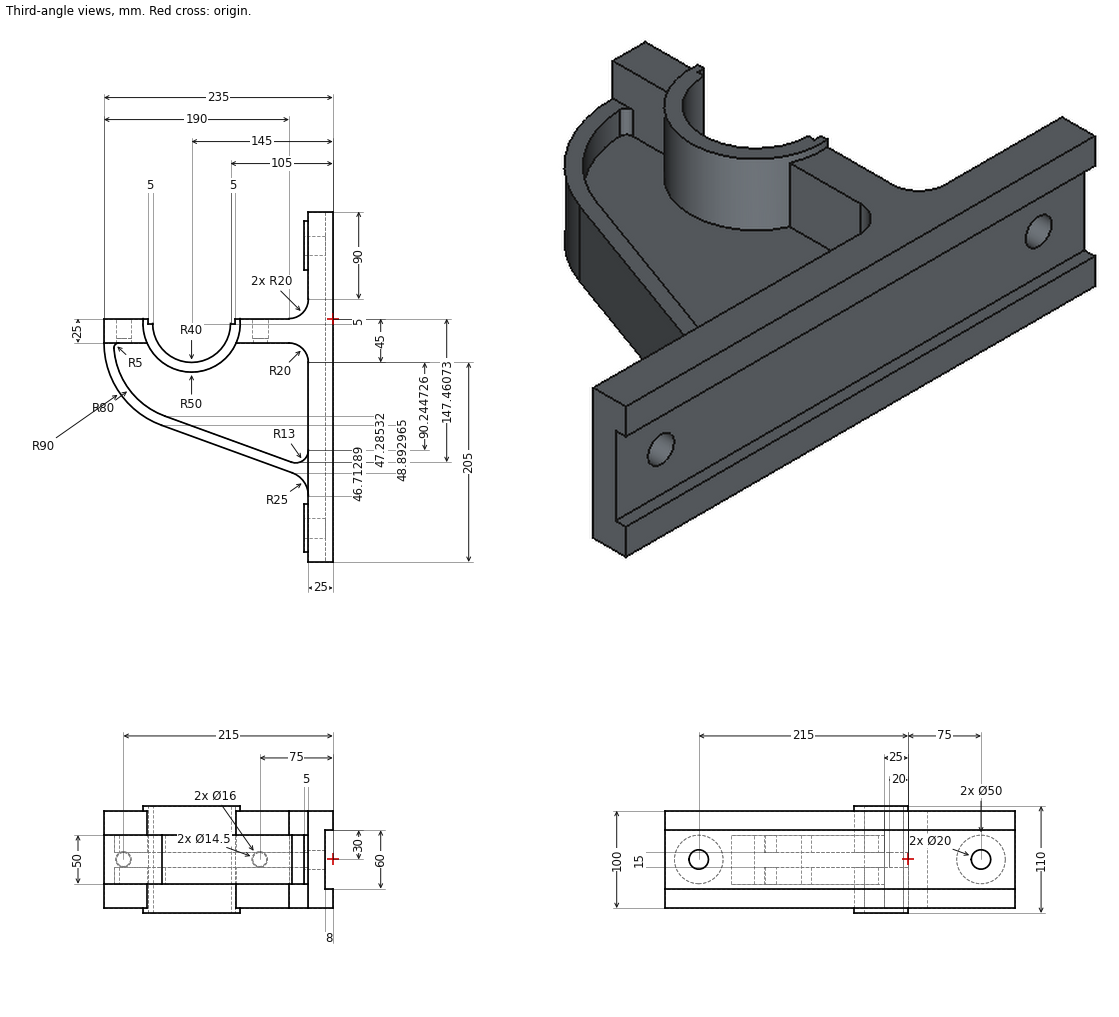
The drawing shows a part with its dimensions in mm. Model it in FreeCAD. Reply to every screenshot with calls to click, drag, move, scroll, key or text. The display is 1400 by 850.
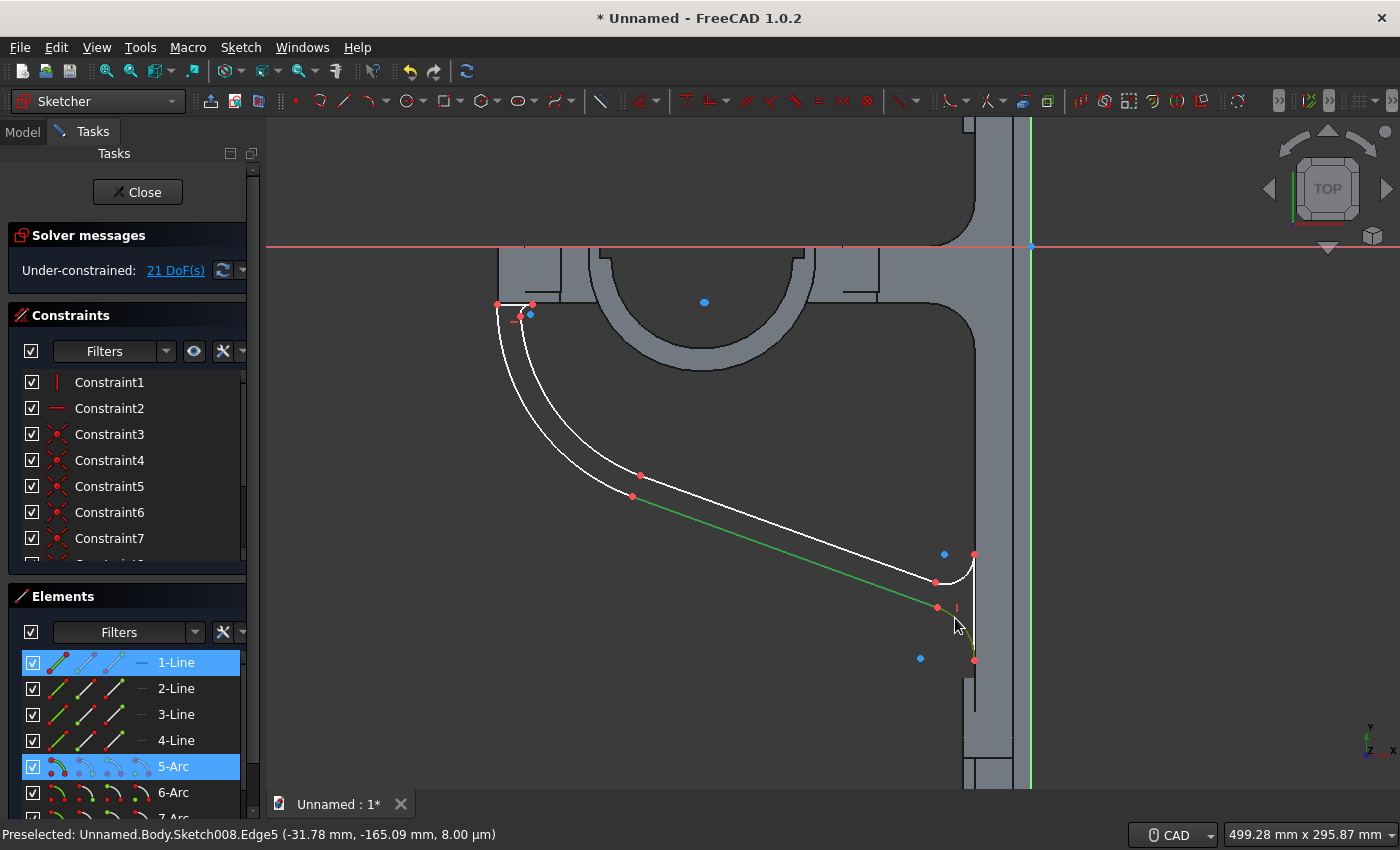
click(796, 102)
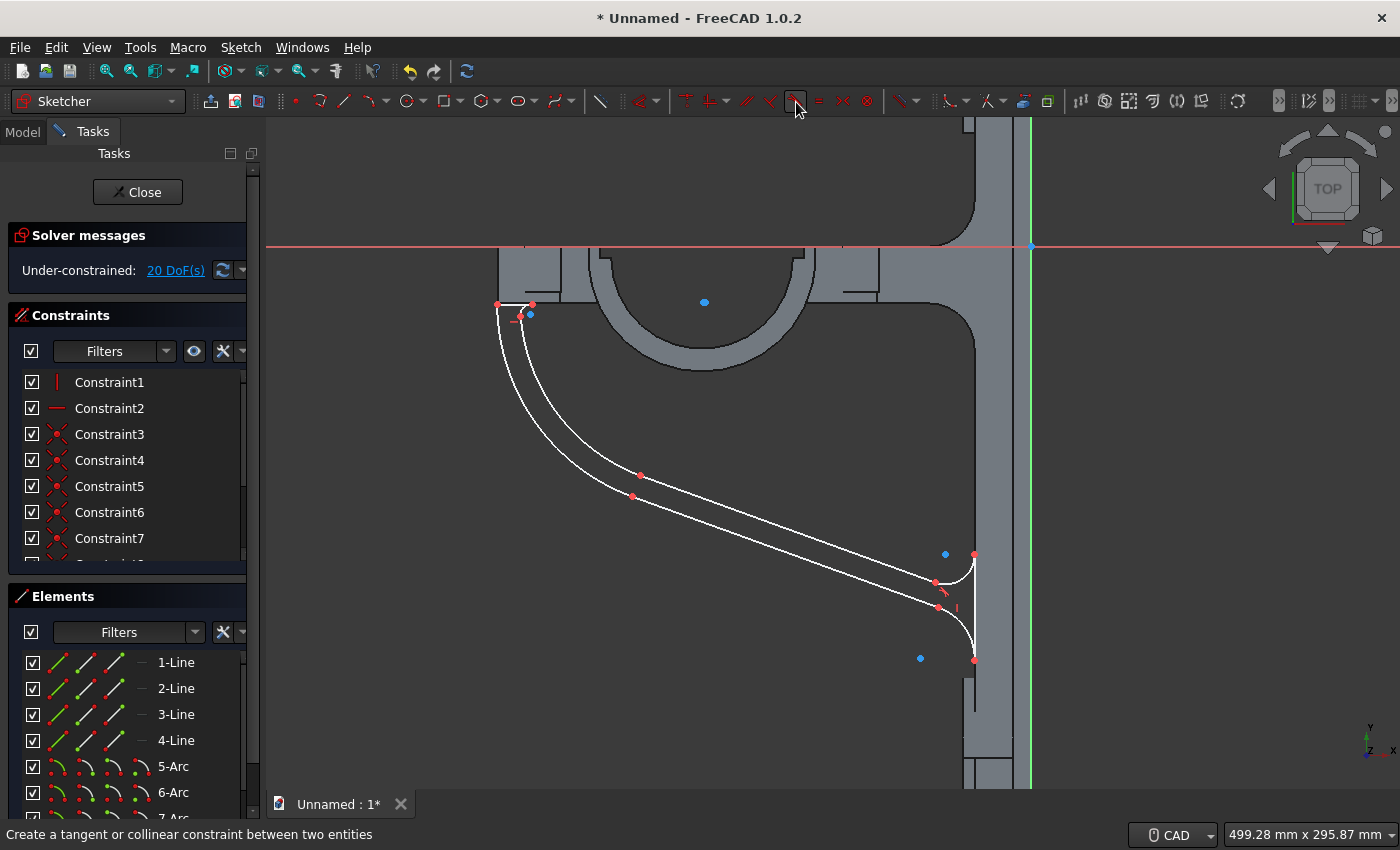
click(975, 586)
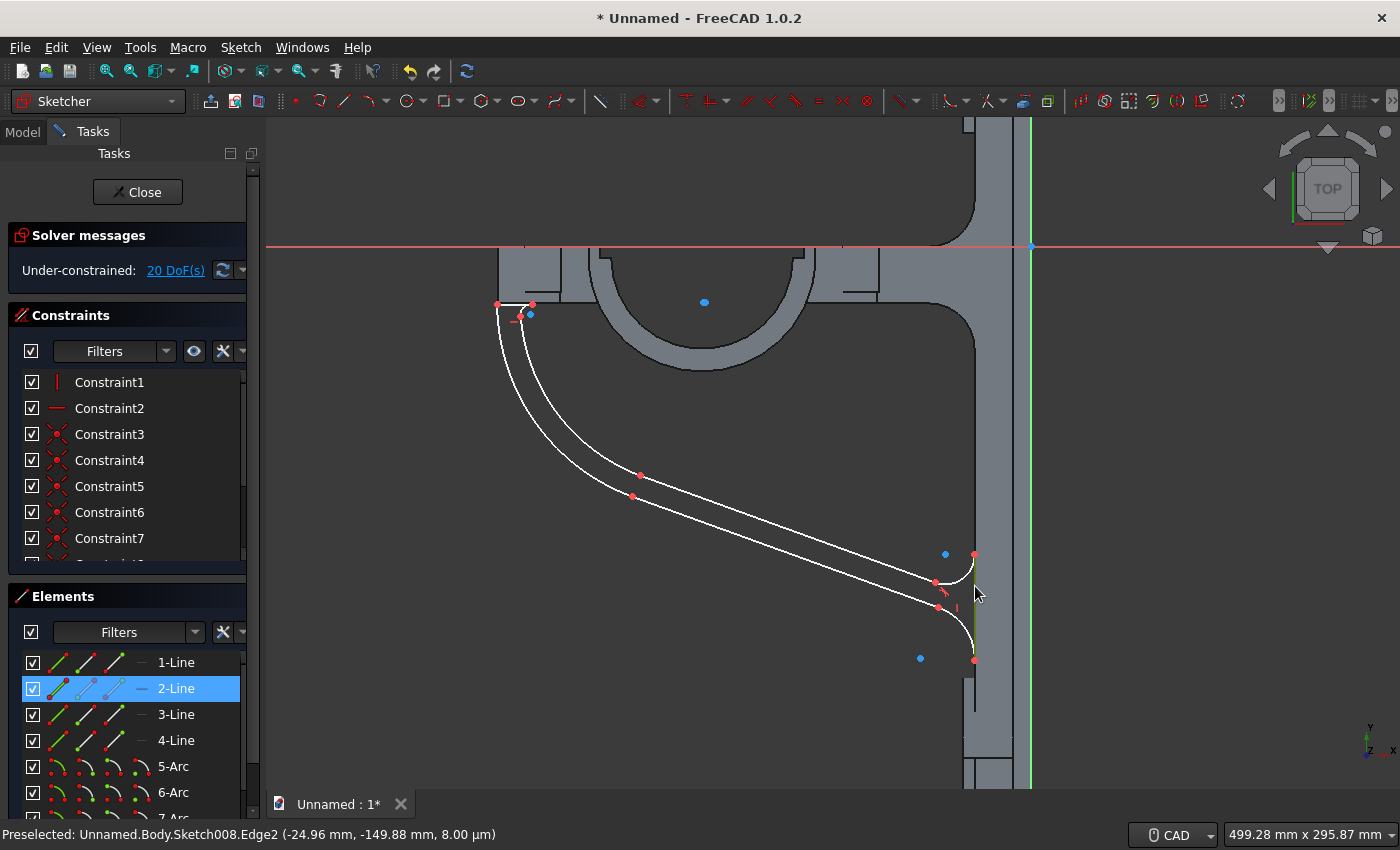
click(956, 618)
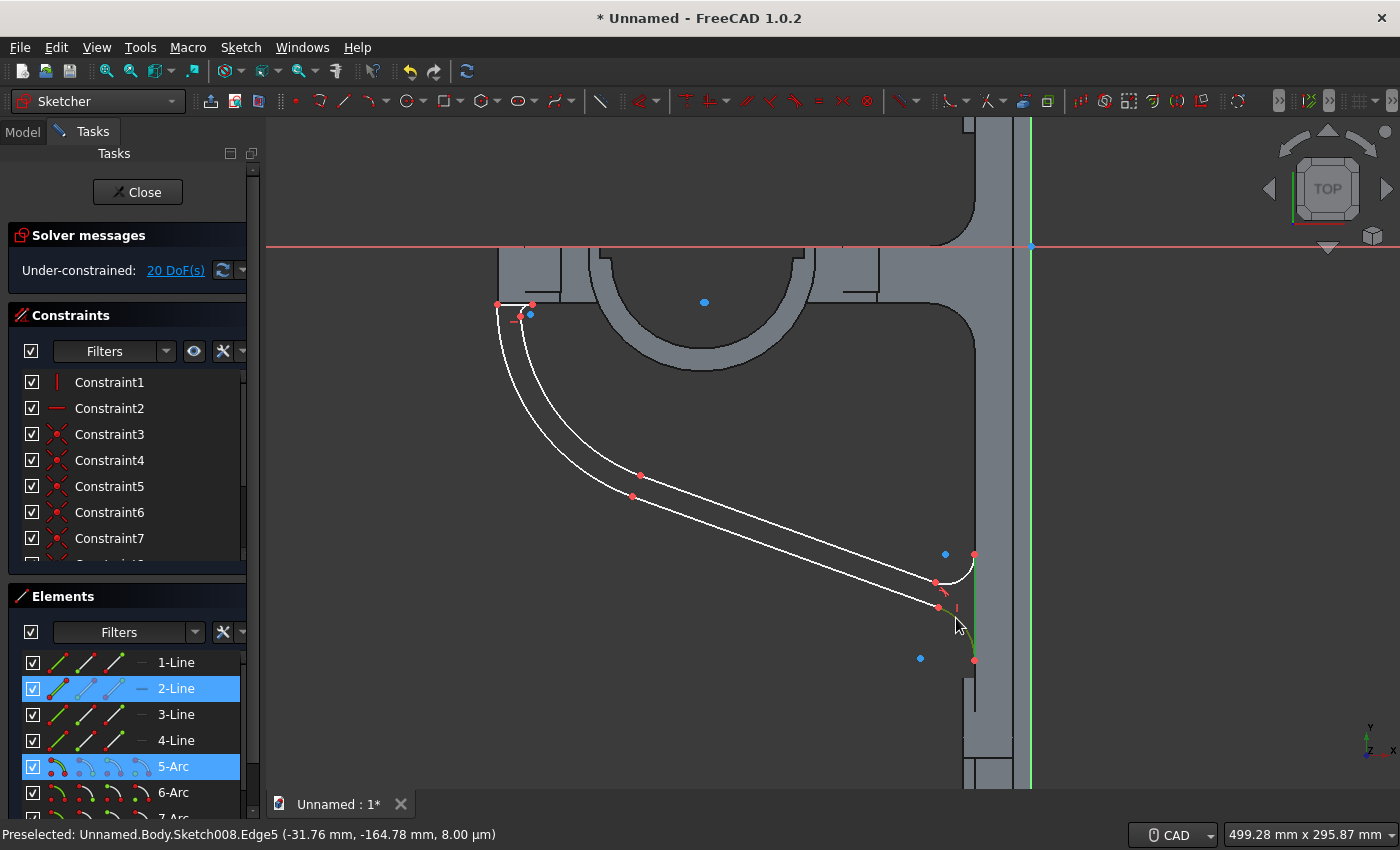
click(796, 102)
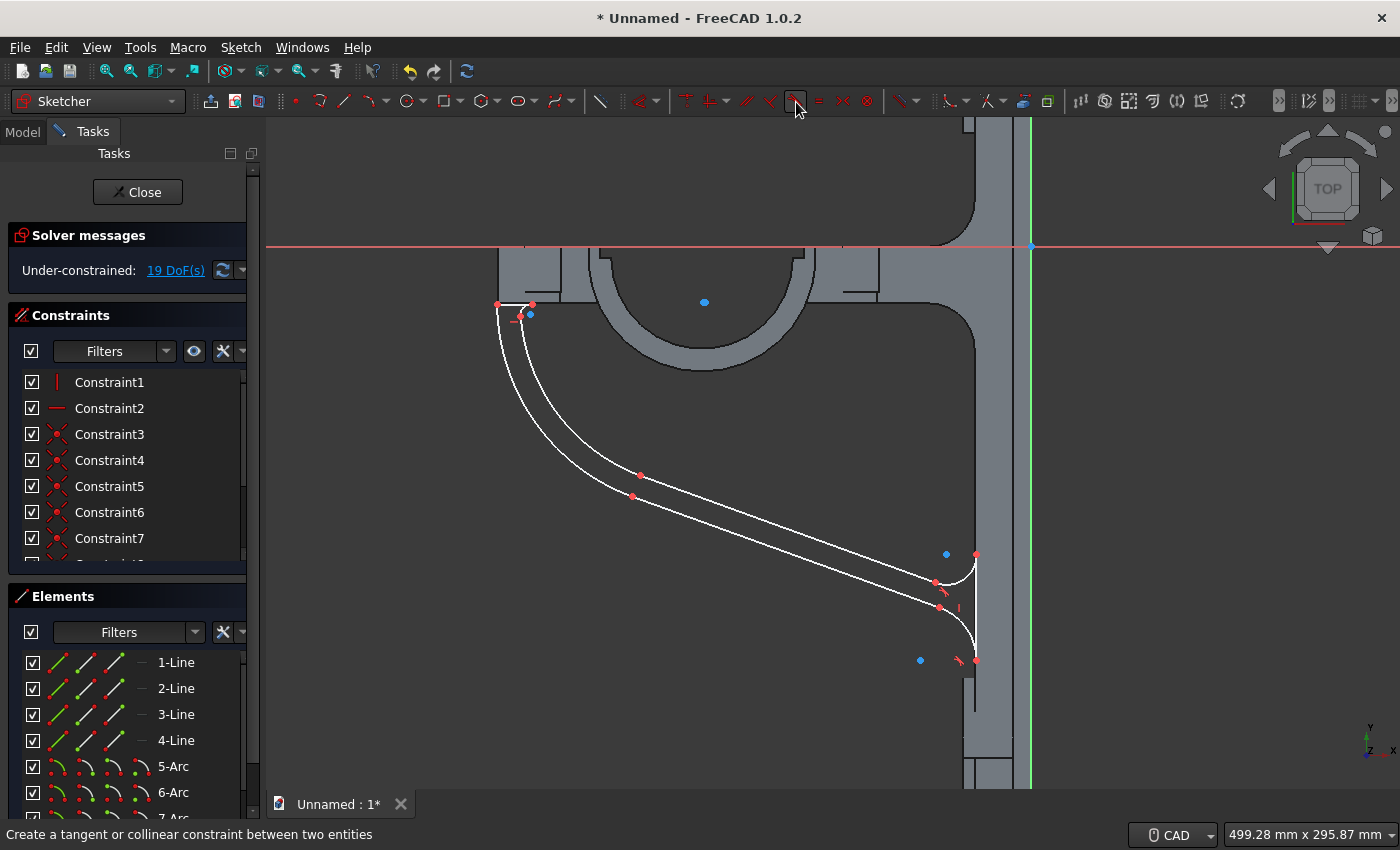
click(976, 586)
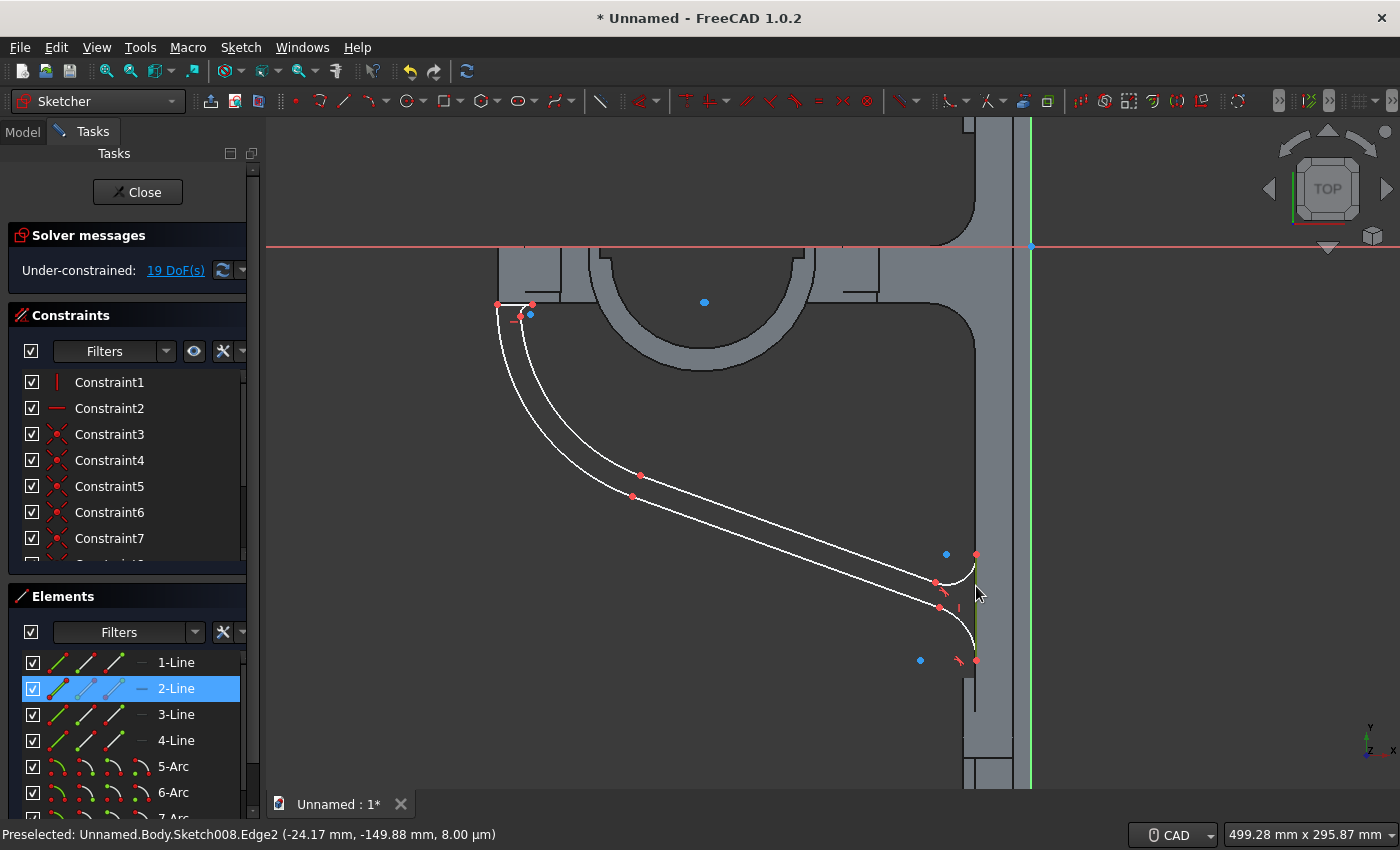
click(953, 584)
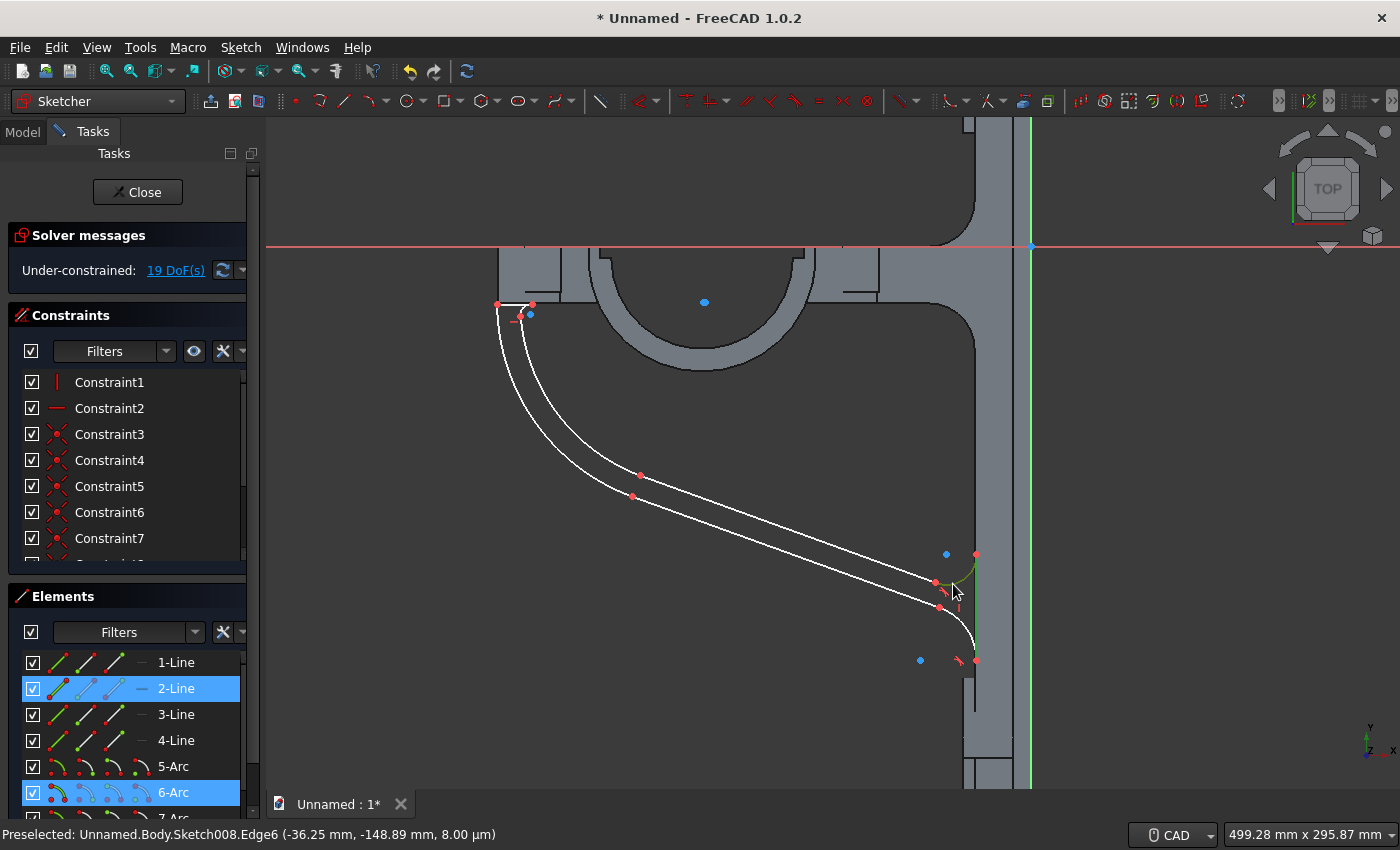
click(796, 102)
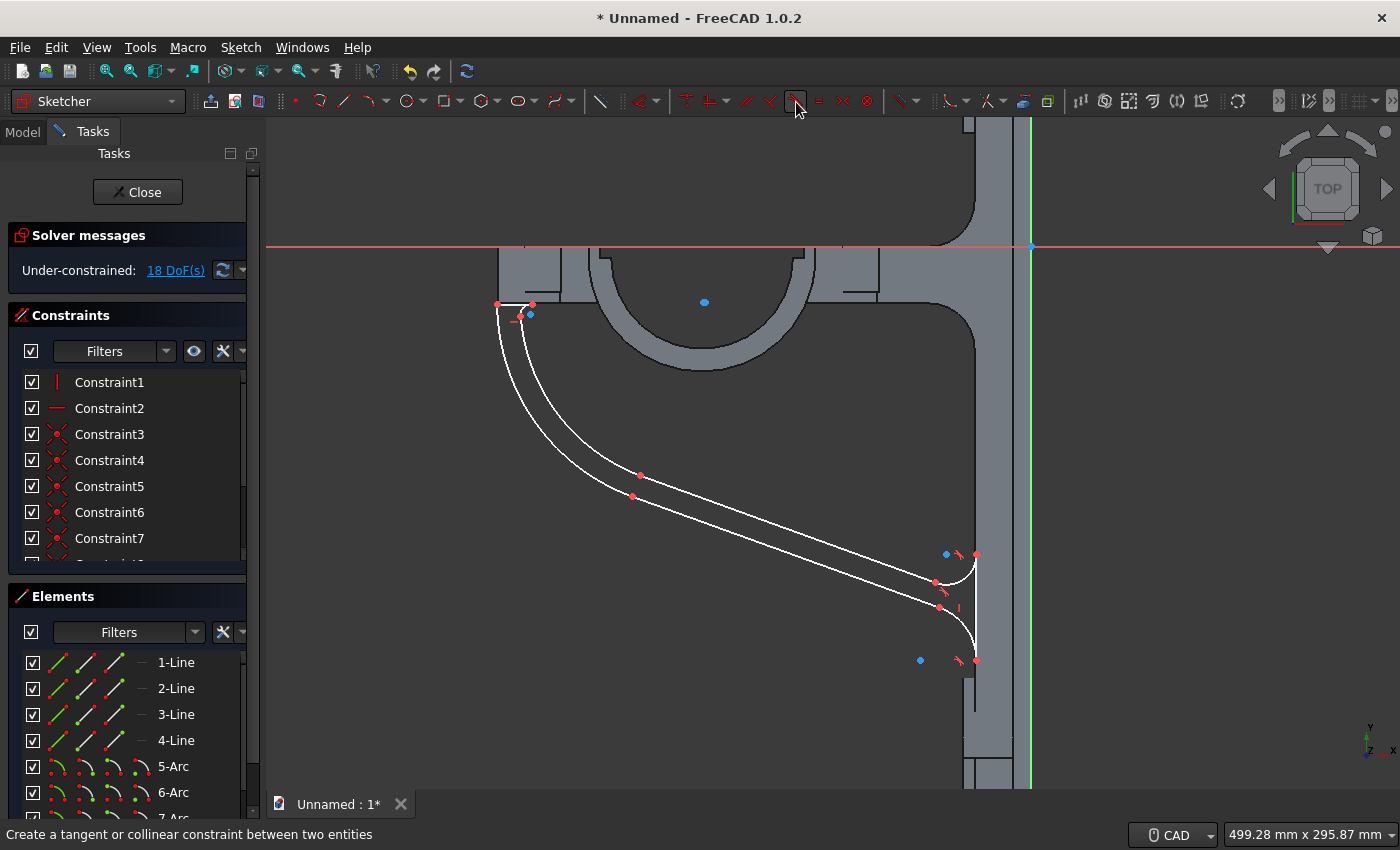
click(847, 551)